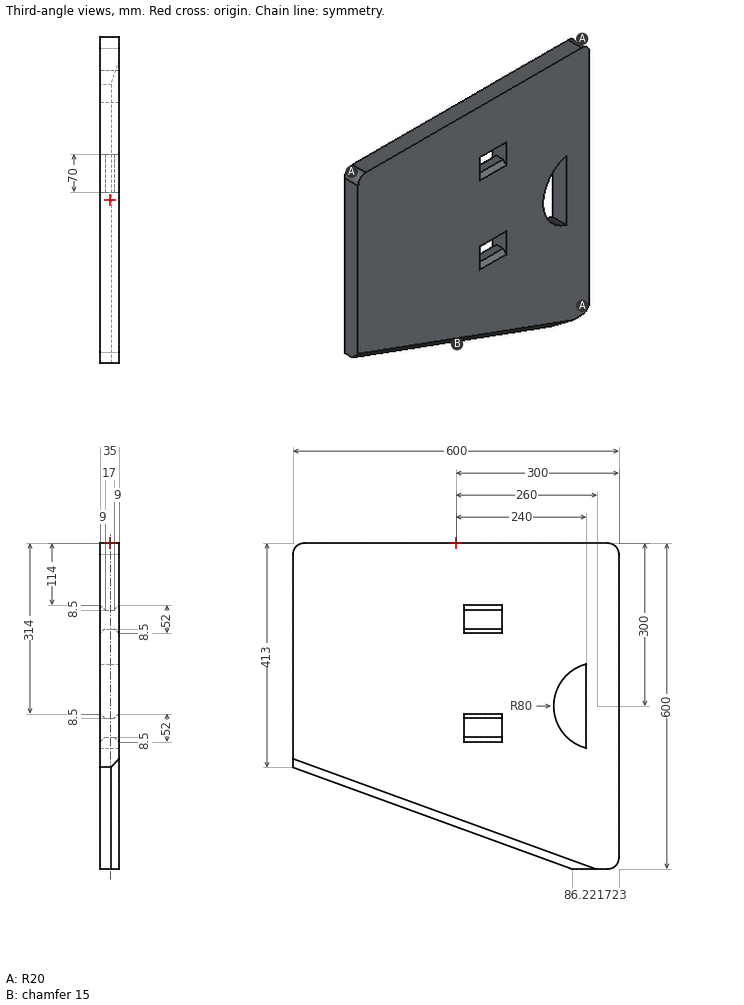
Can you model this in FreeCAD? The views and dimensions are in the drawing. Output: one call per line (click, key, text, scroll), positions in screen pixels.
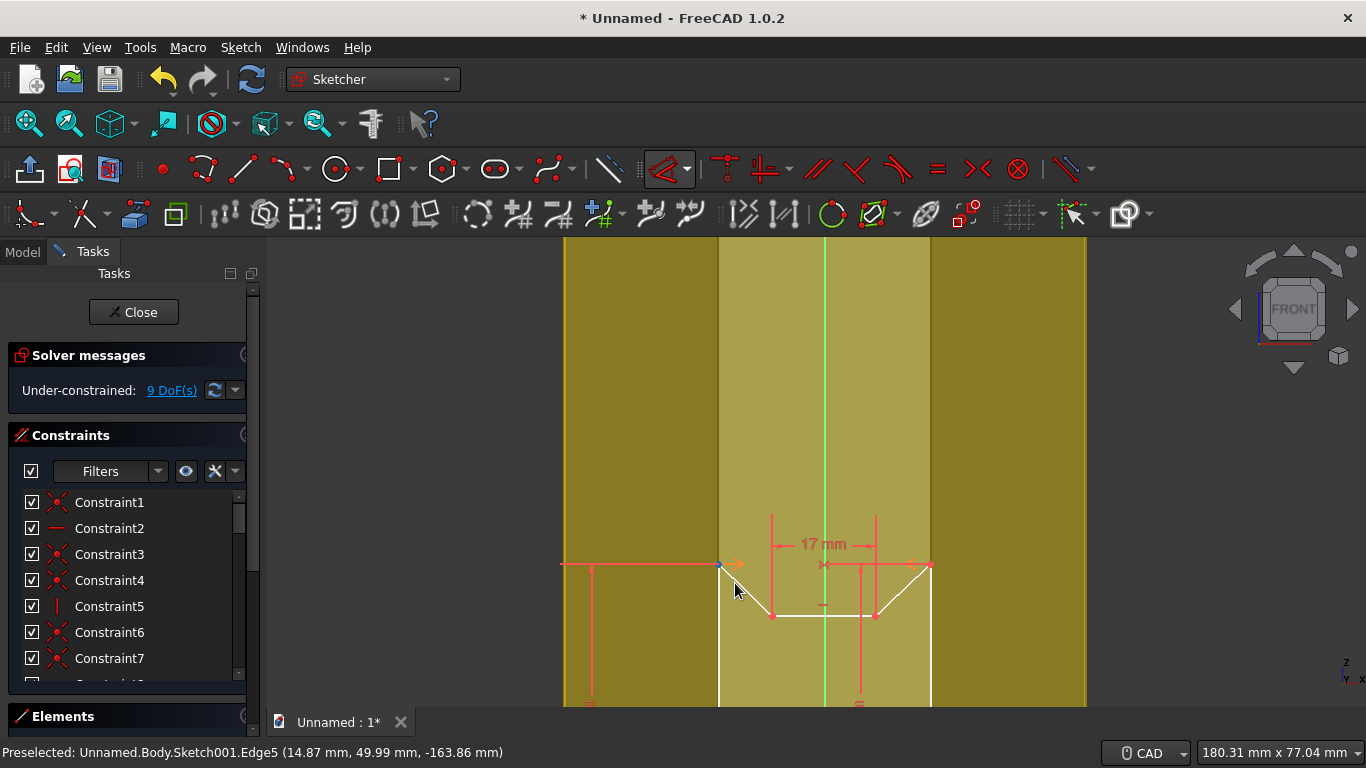
click(735, 580)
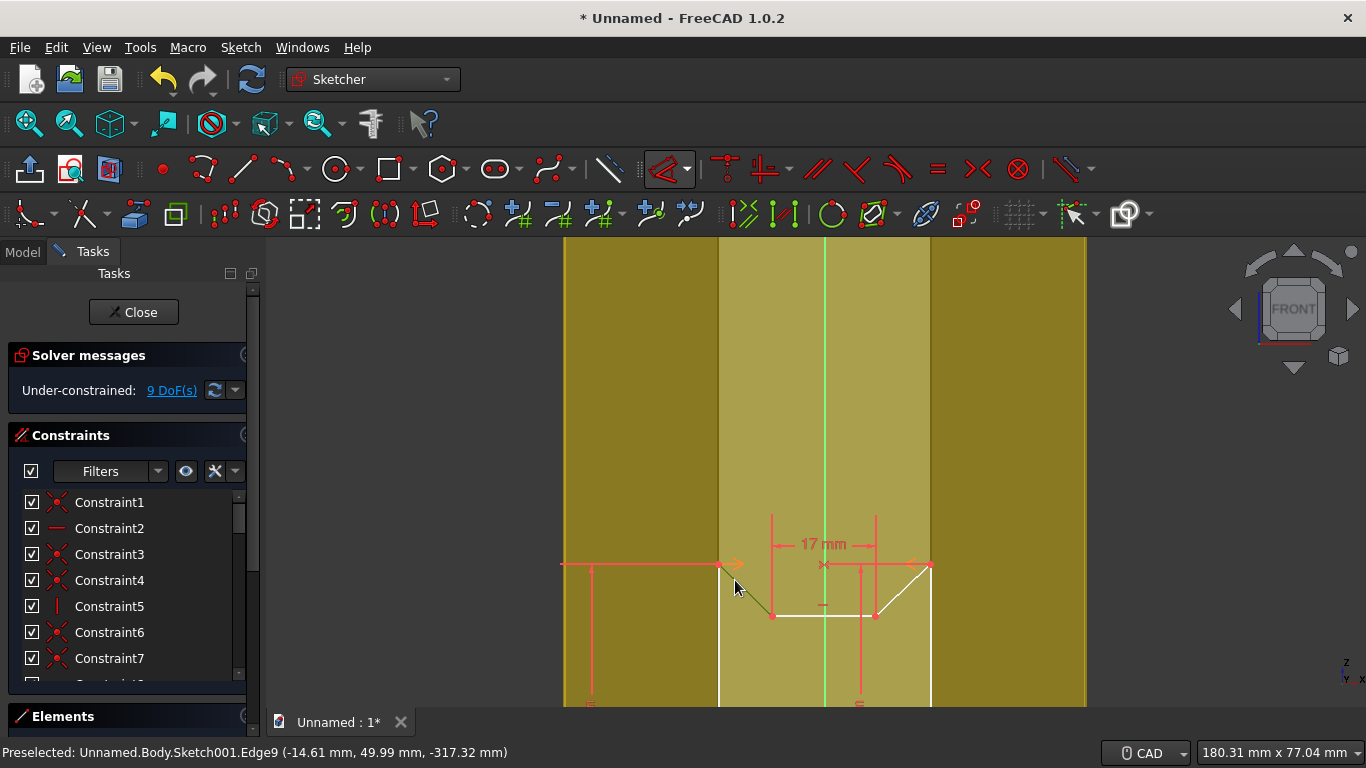
click(690, 170)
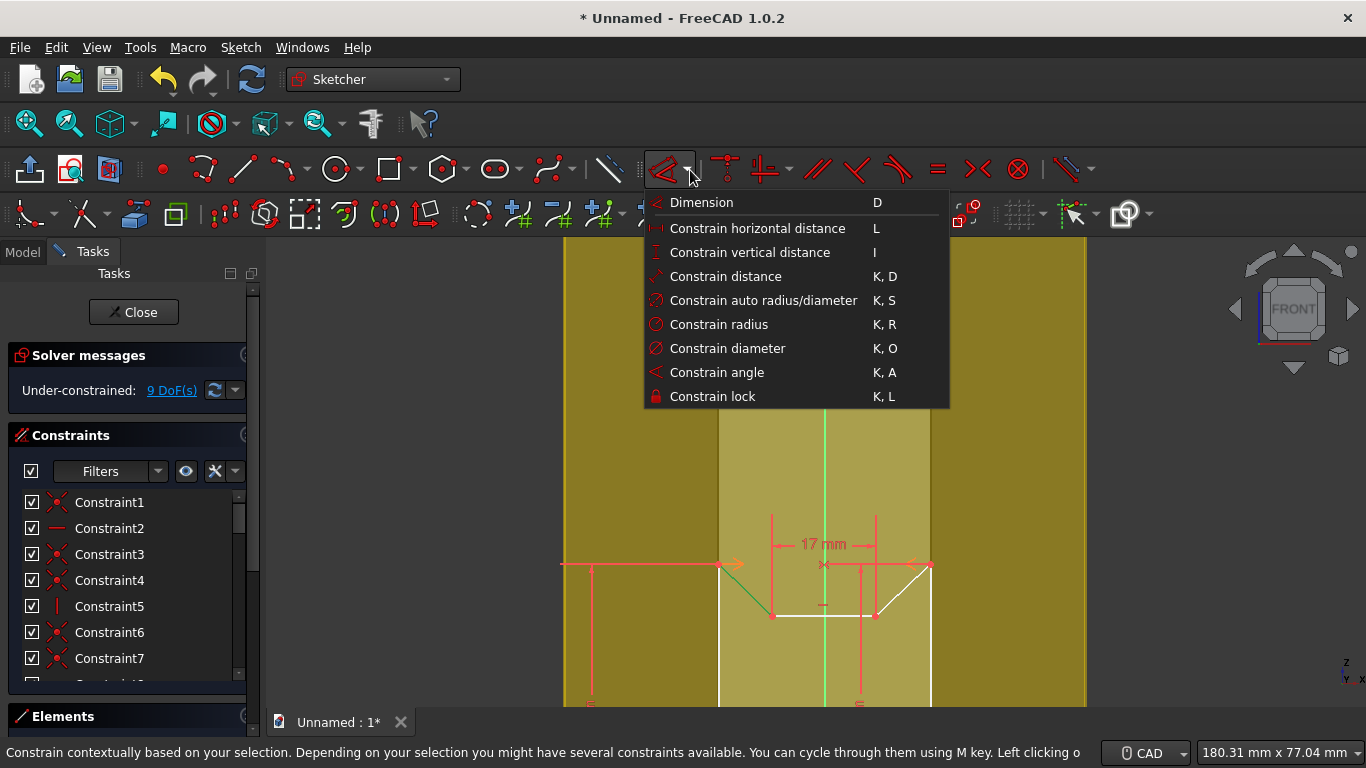
click(797, 228)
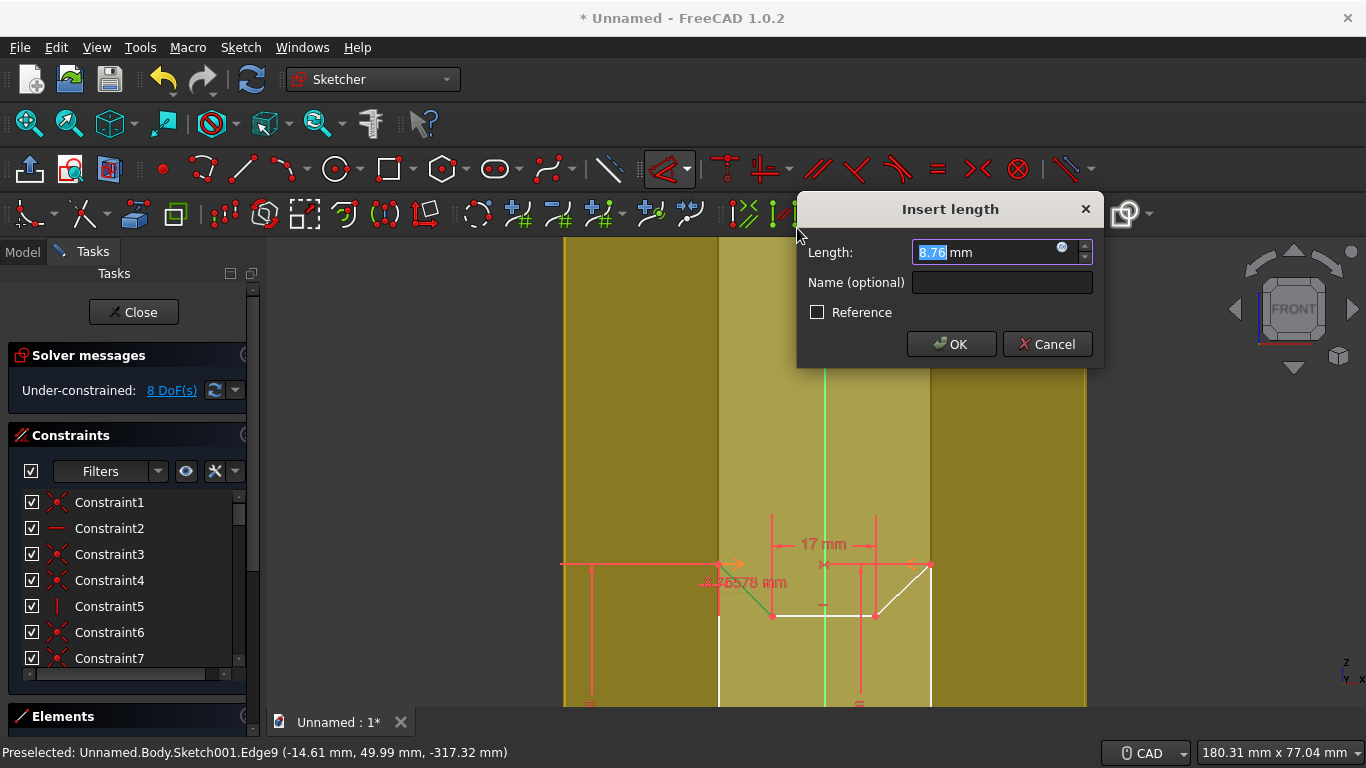
text(9)
key(Return)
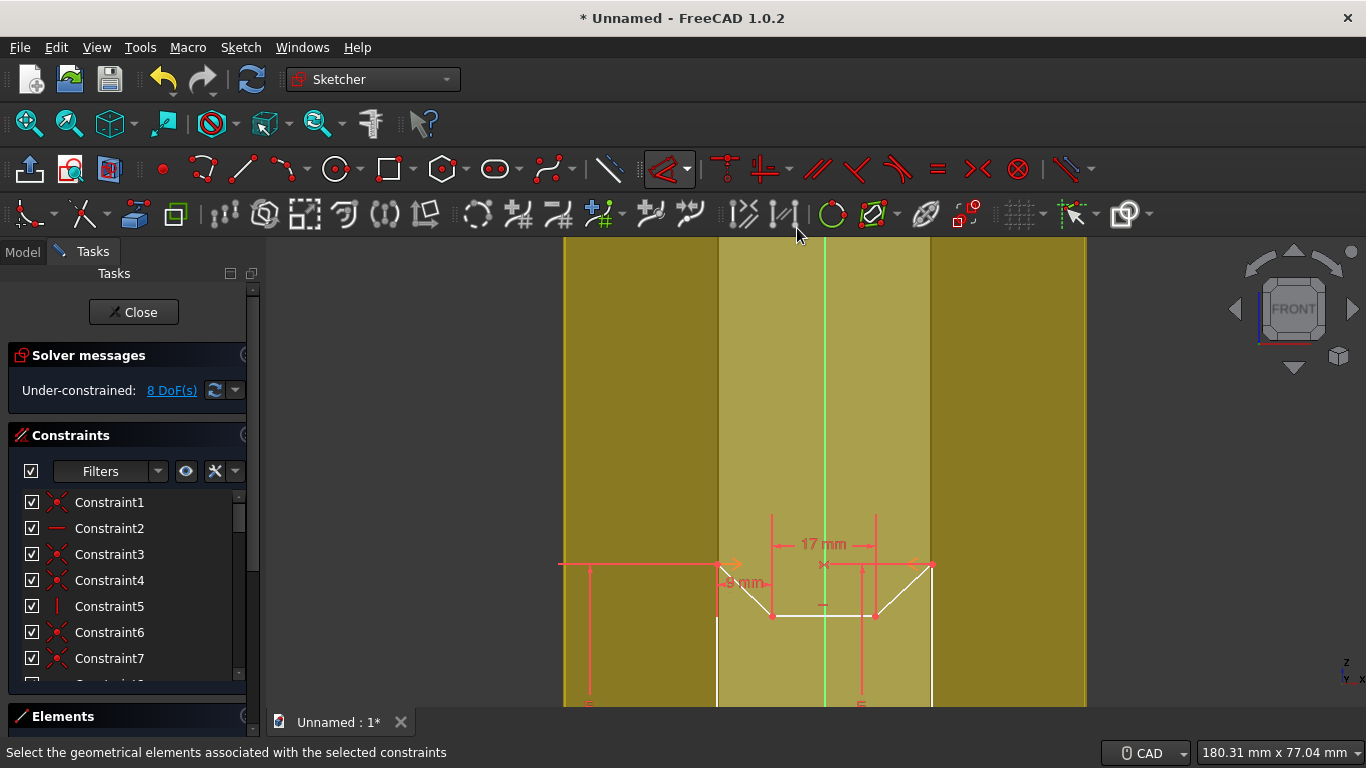
click(893, 600)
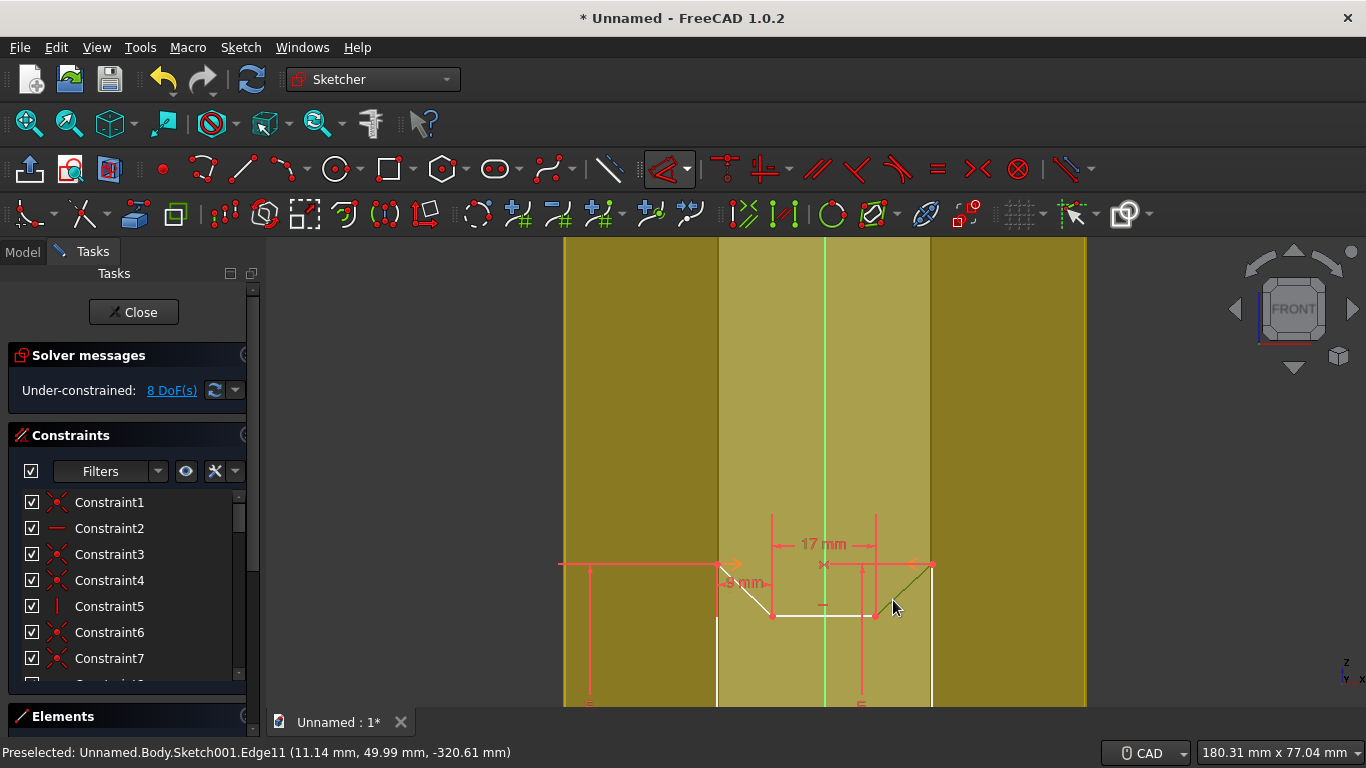
key(l)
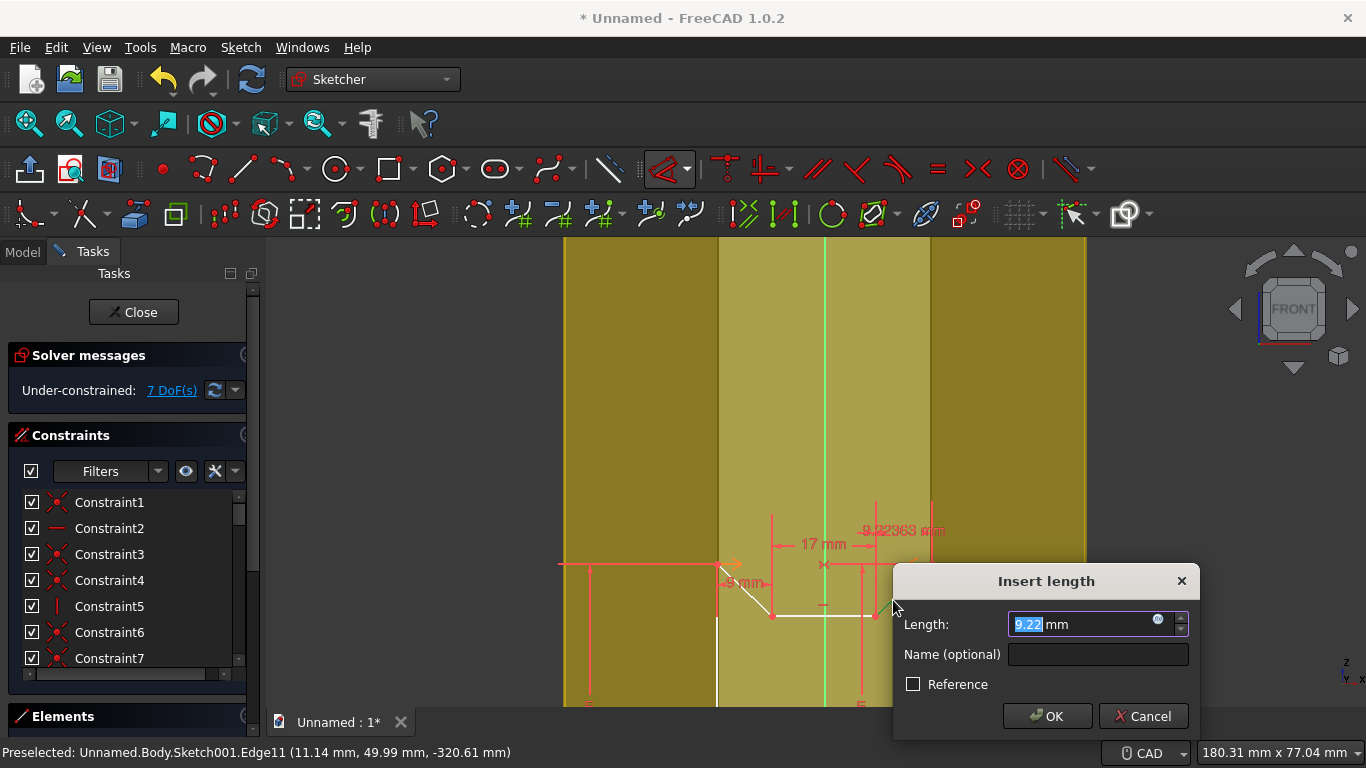
text(9)
key(Return)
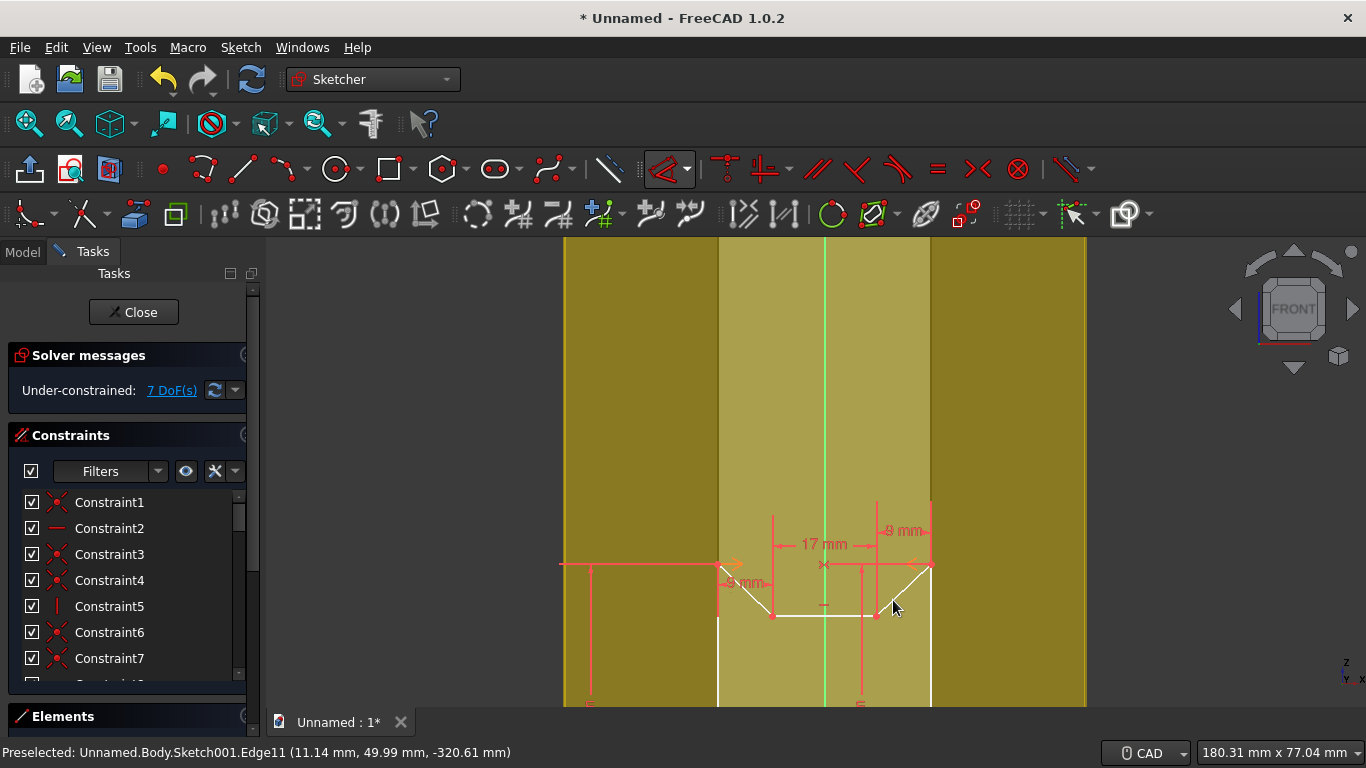
scroll(735, 583, down, 10)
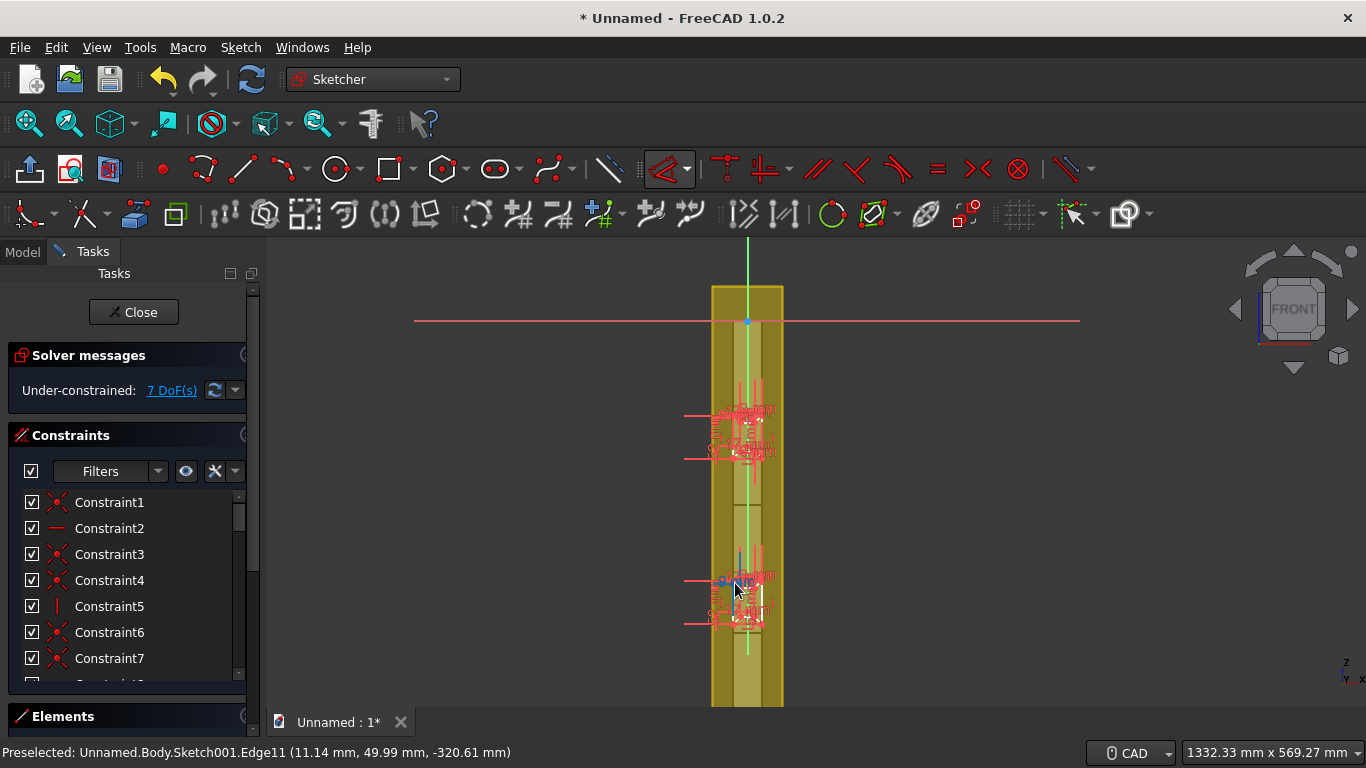
scroll(760, 622, up, 10)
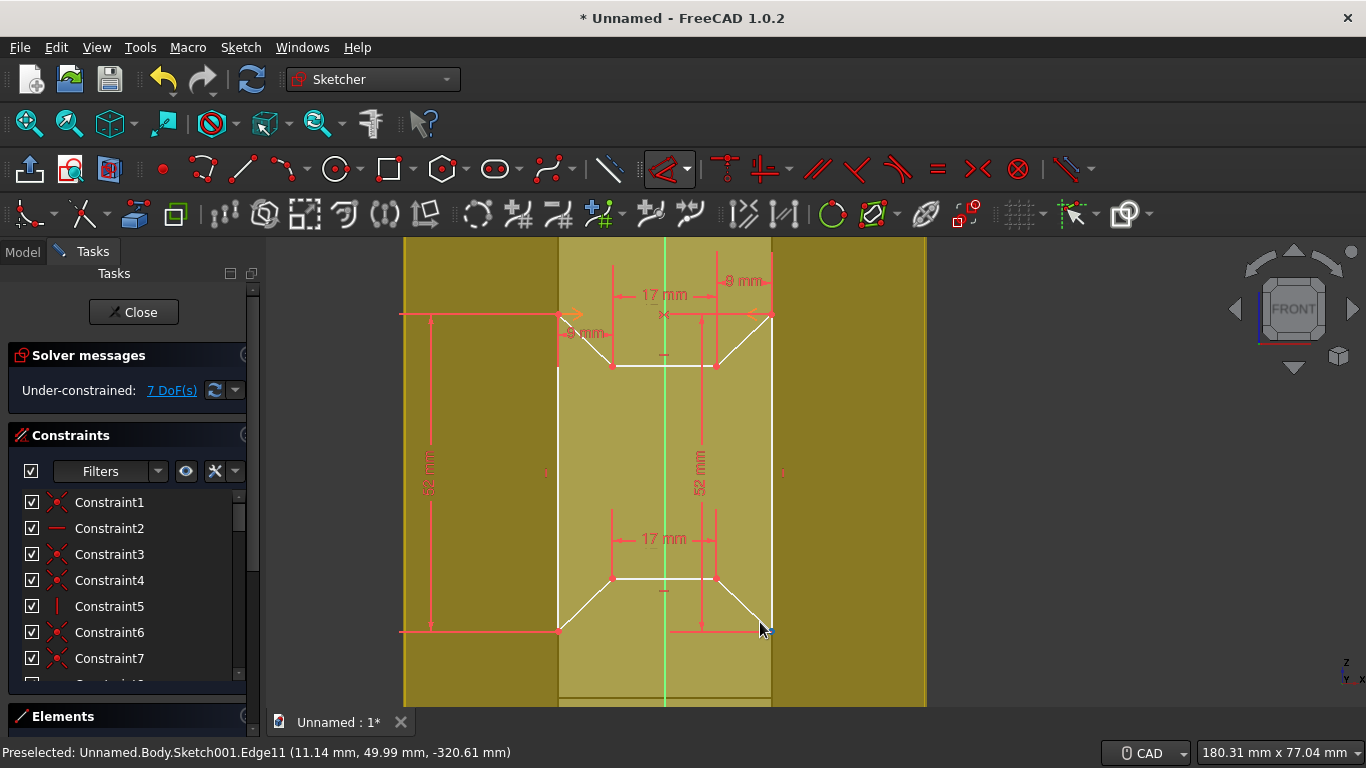
click(755, 616)